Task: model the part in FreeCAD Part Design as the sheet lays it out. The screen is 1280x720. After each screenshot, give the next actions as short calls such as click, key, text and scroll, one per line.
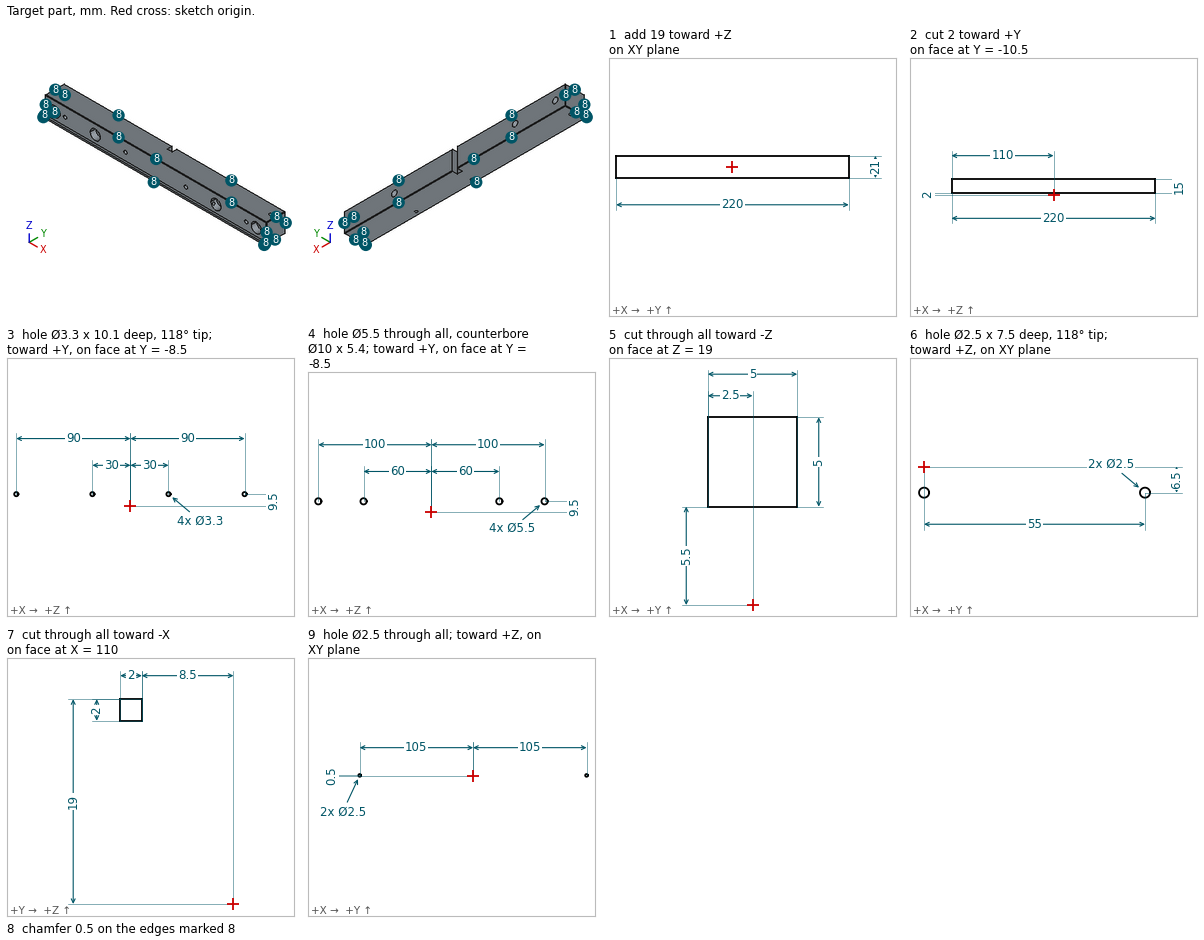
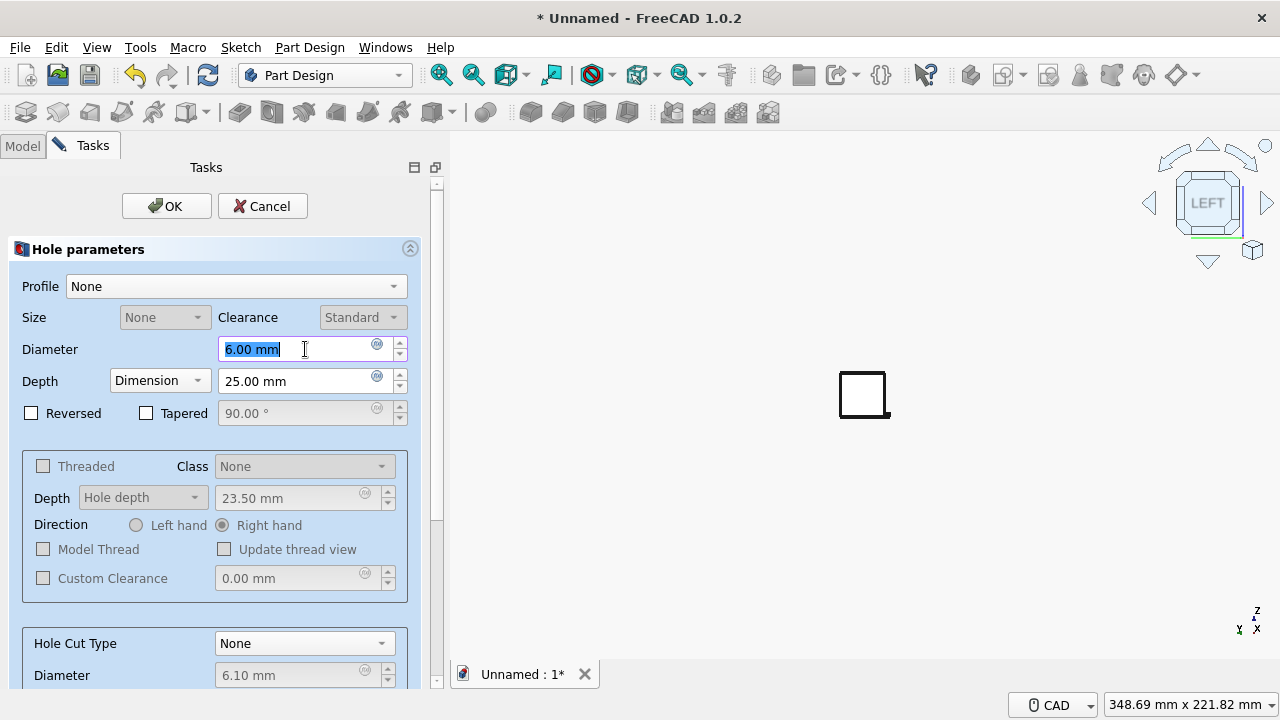
text(2.5)
key(Tab)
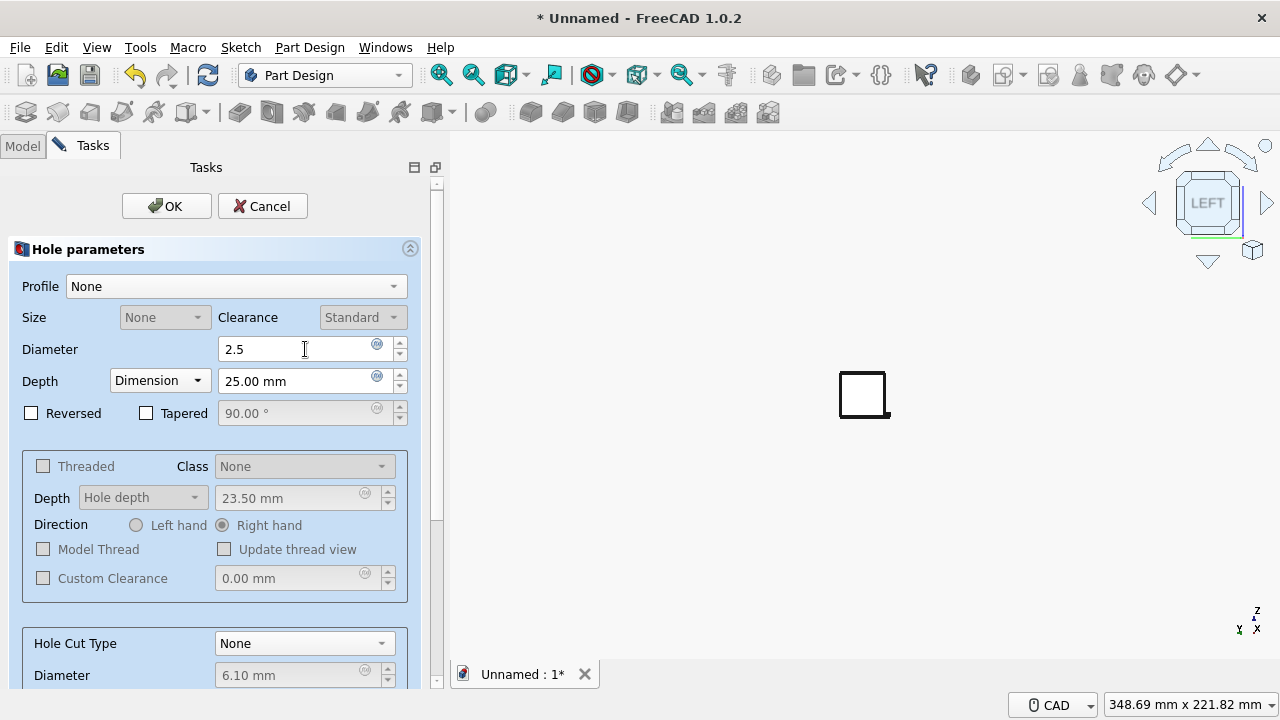
click(161, 380)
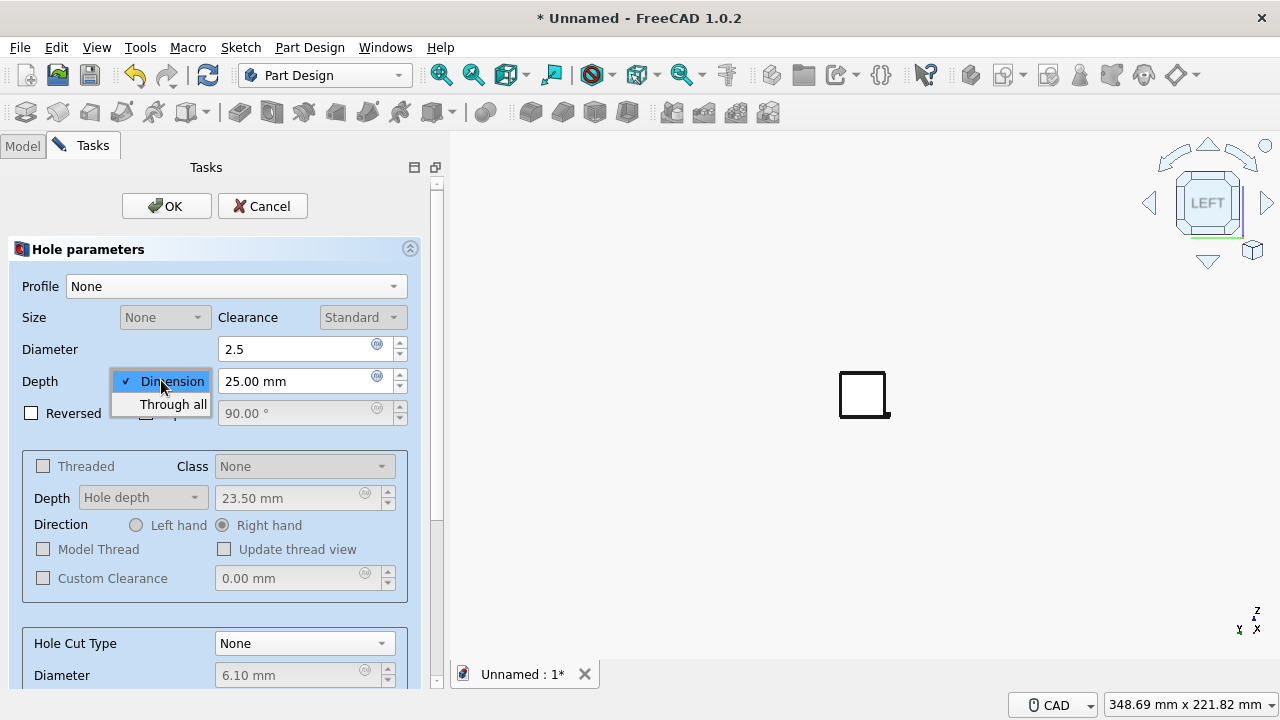
click(160, 404)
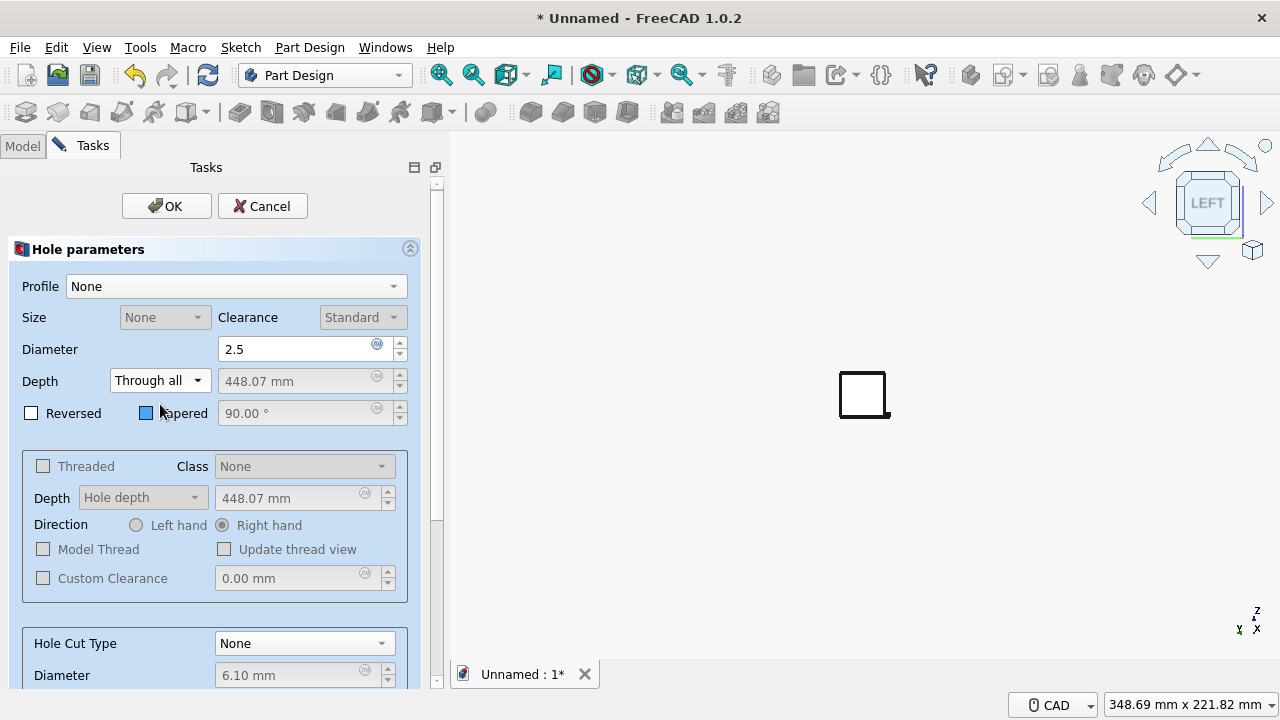
click(30, 413)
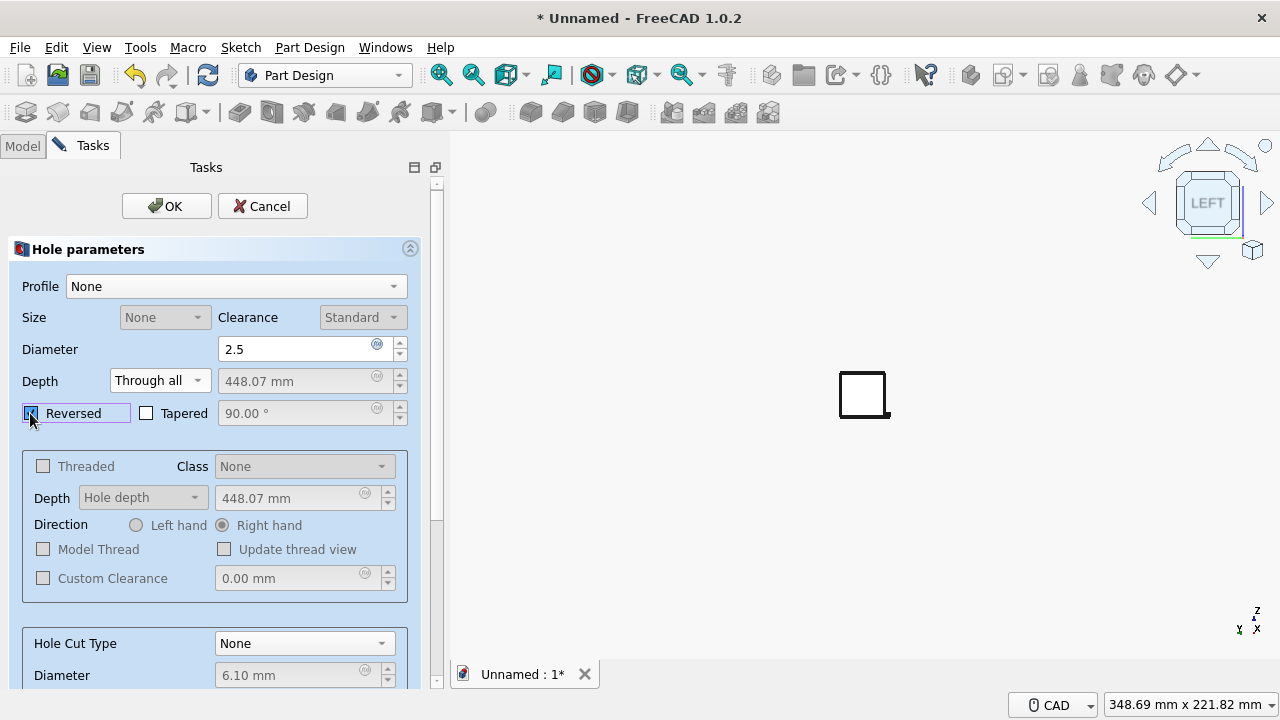
click(167, 206)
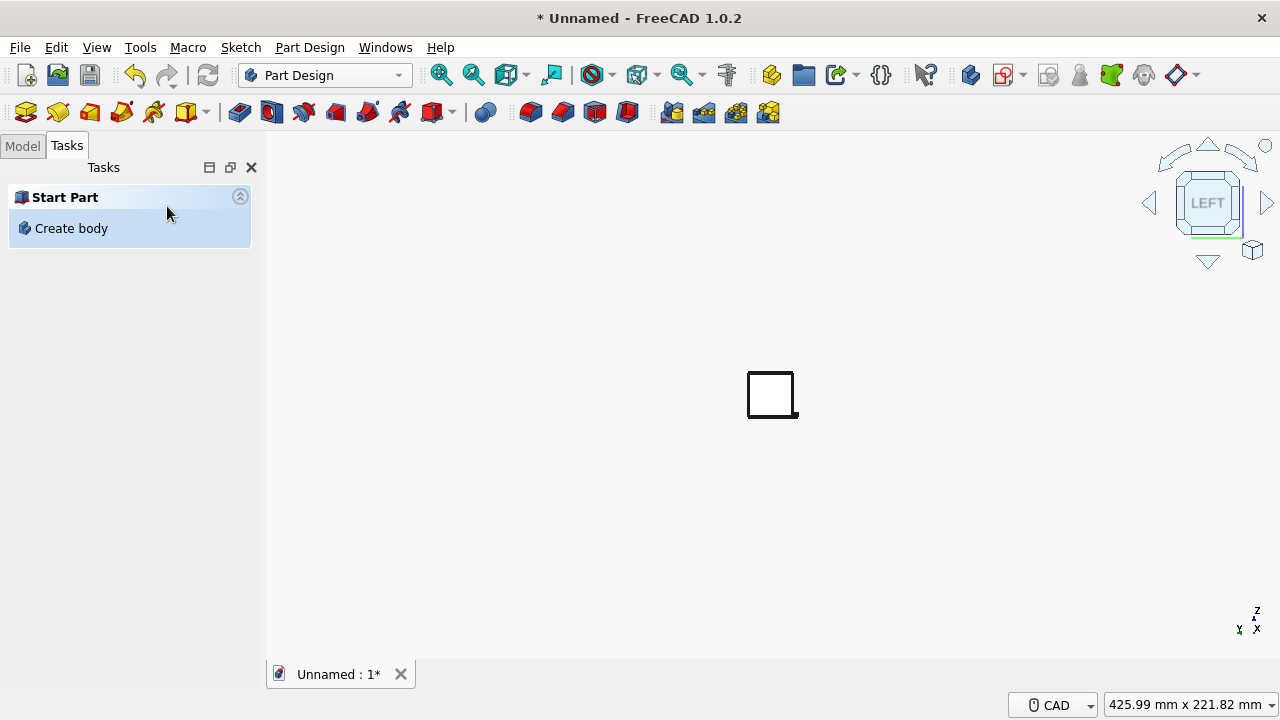
key(0)